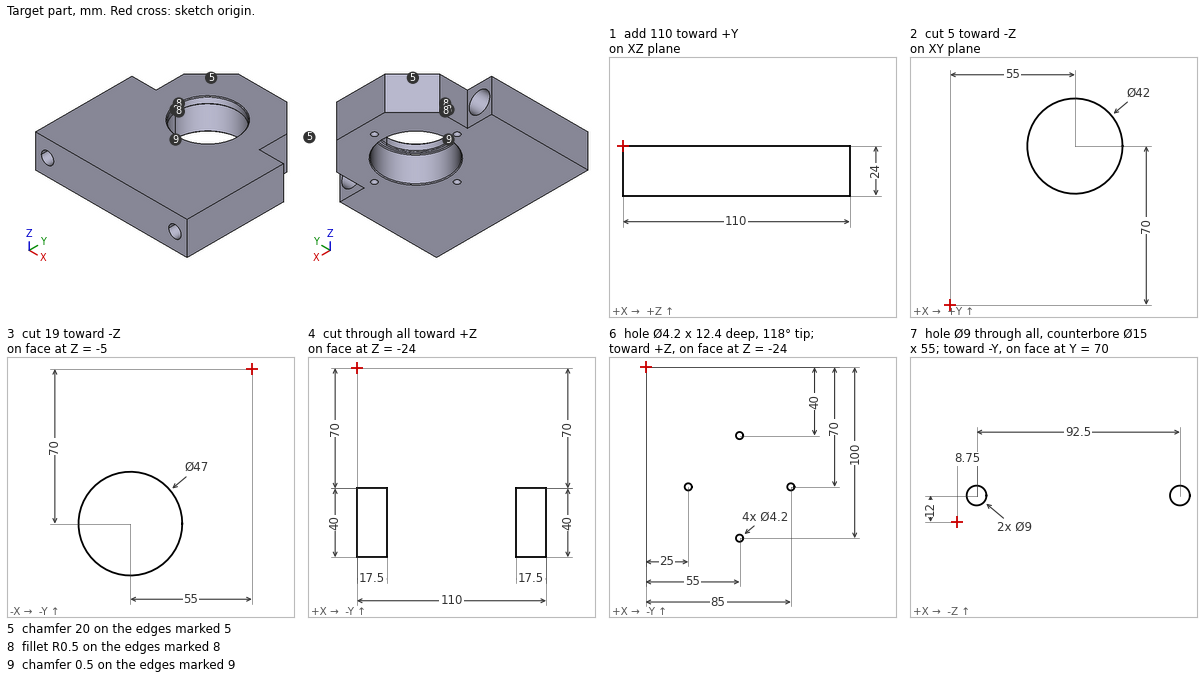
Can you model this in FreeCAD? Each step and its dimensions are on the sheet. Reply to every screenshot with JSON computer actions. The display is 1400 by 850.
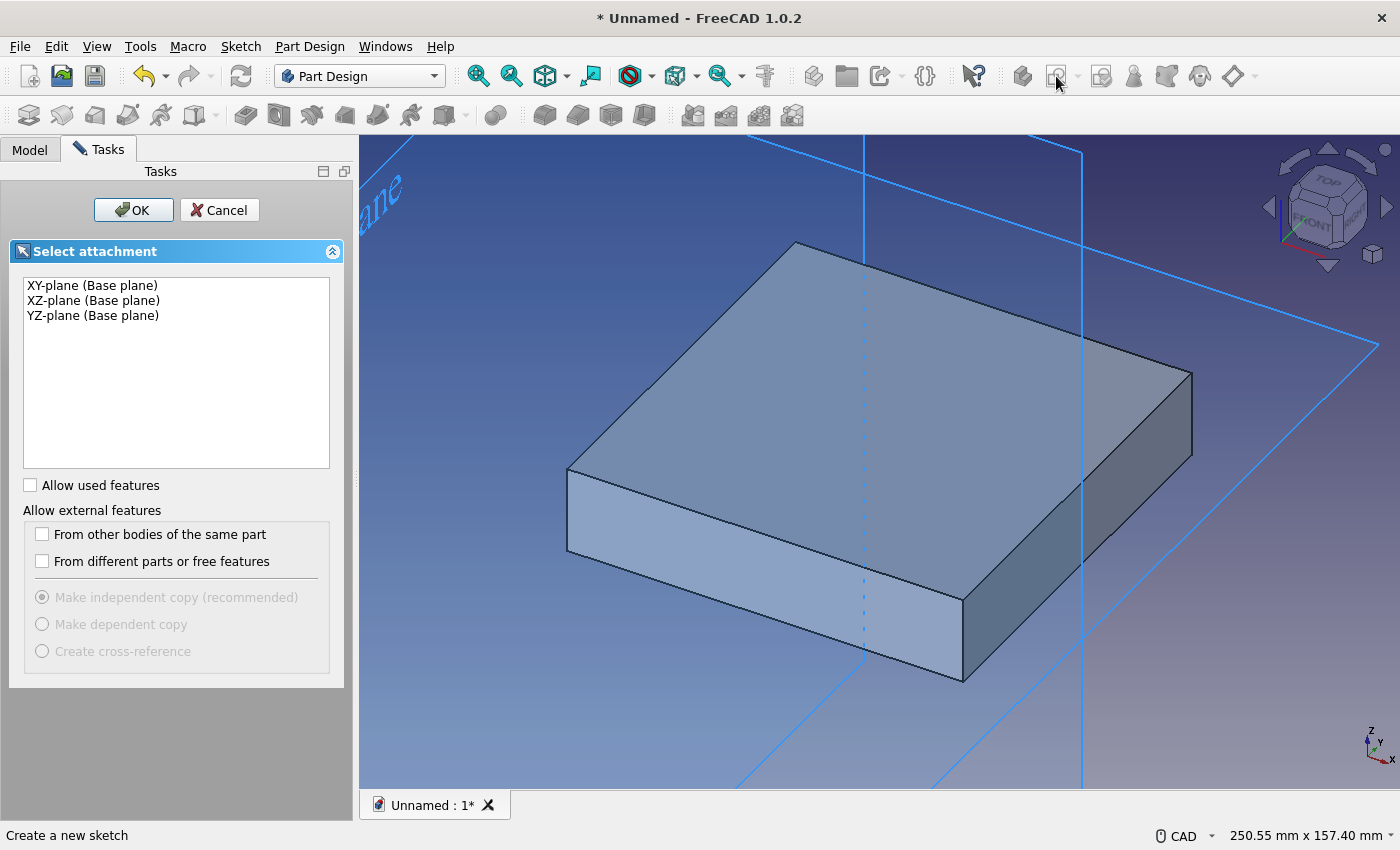
{"action": "left_click", "coordinate": [84, 286]}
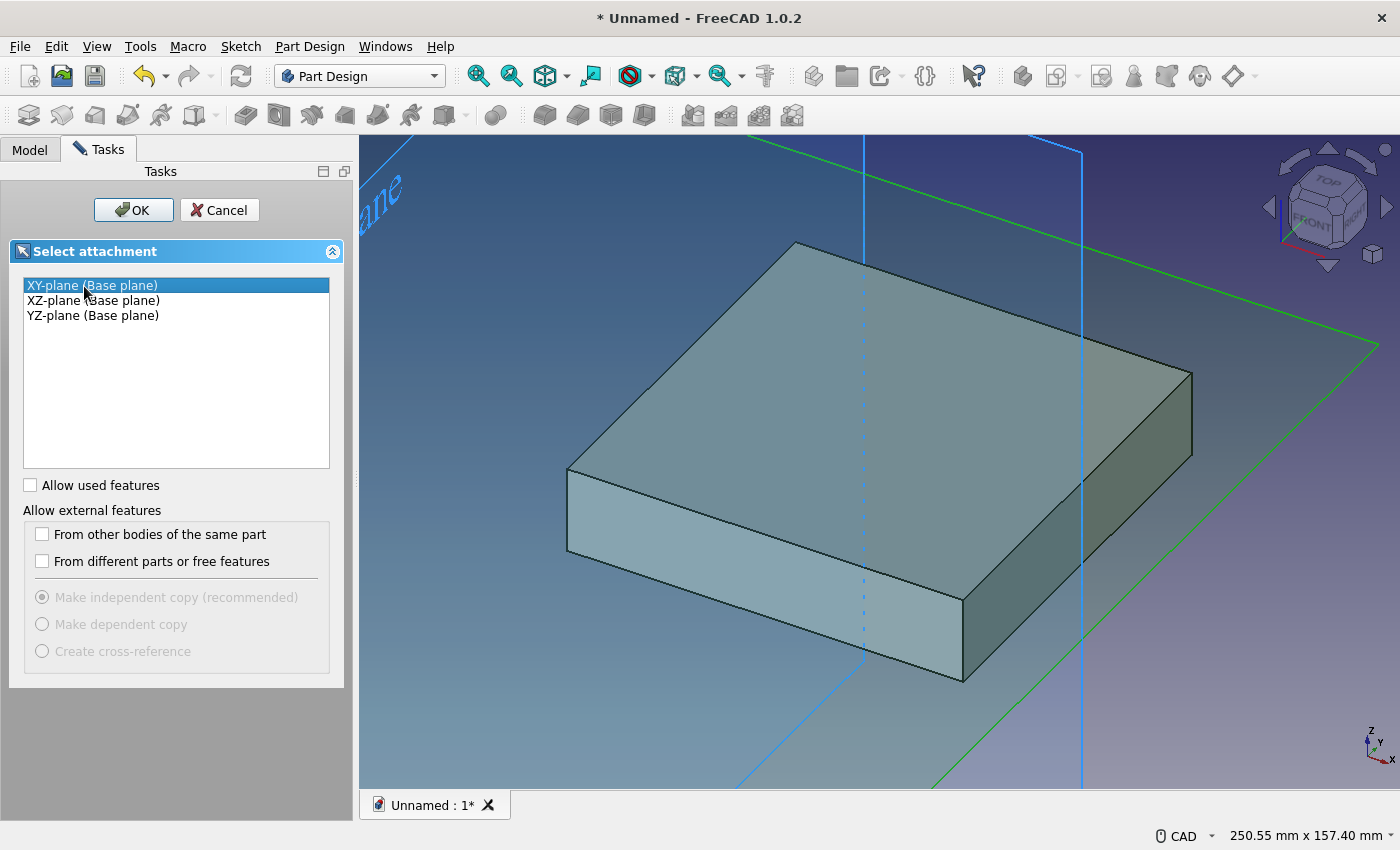
{"action": "left_click", "coordinate": [134, 210]}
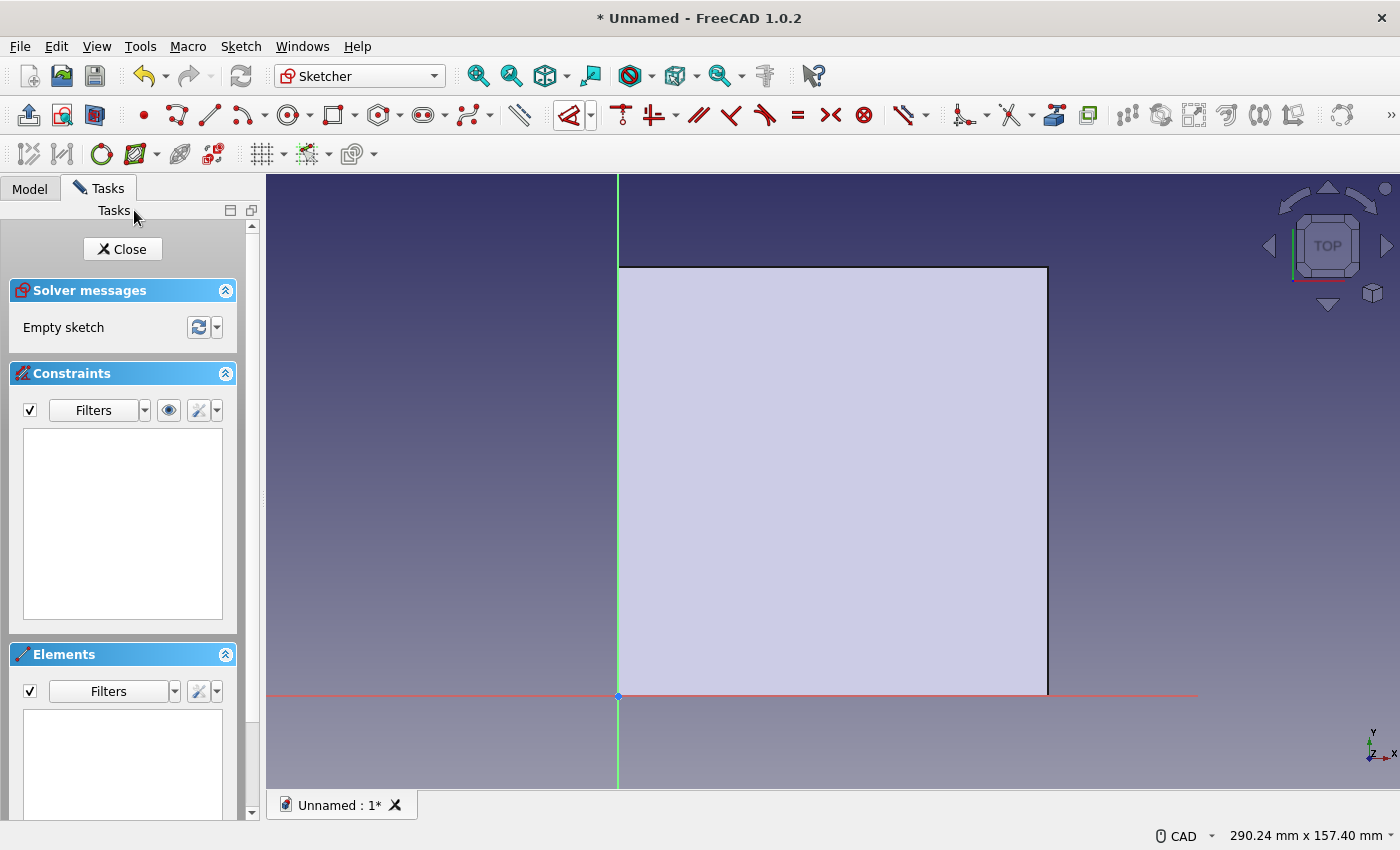
{"action": "left_click", "coordinate": [288, 116]}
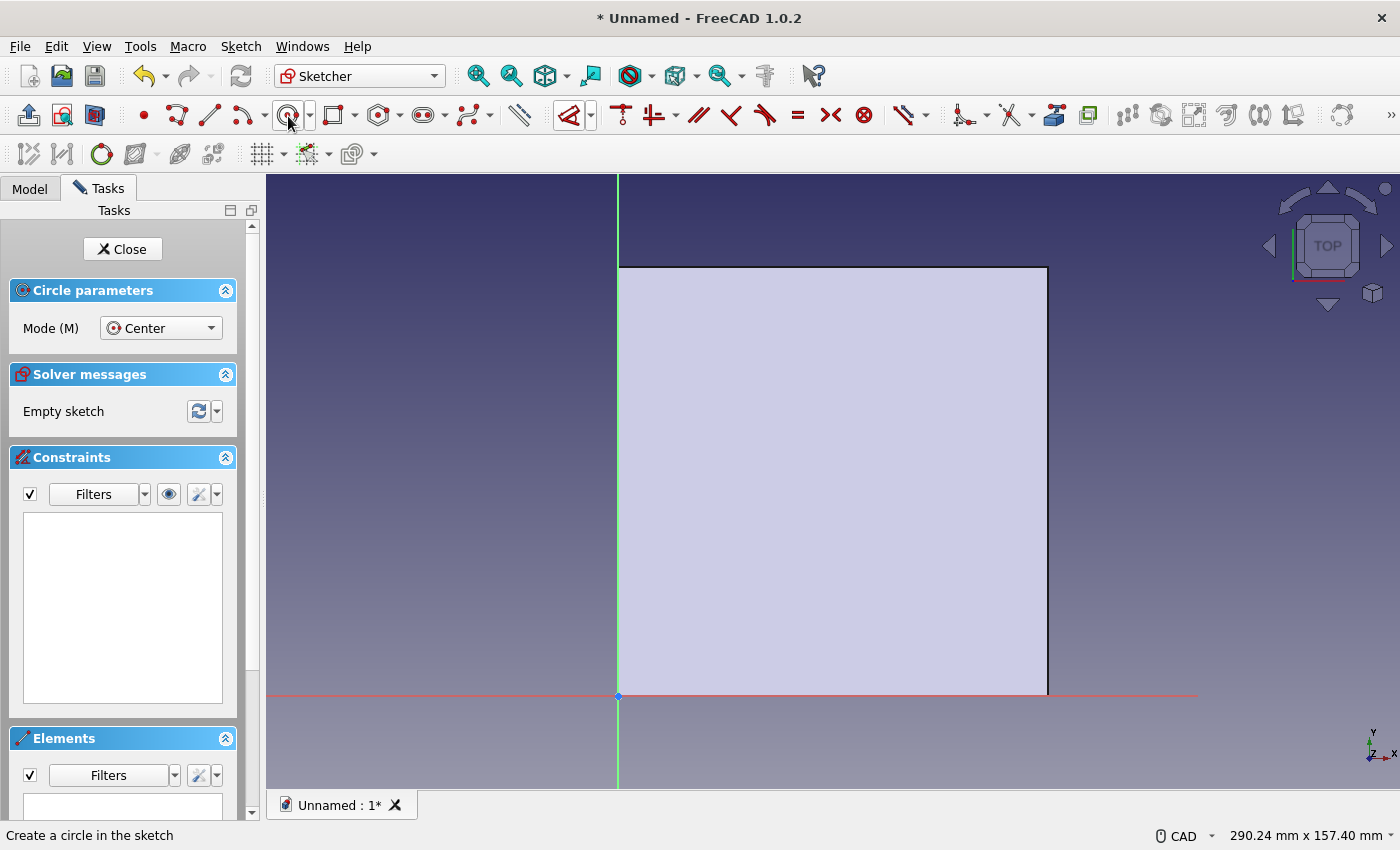
{"action": "left_click", "coordinate": [833, 423]}
{"action": "mouse_move", "coordinate": [891, 365]}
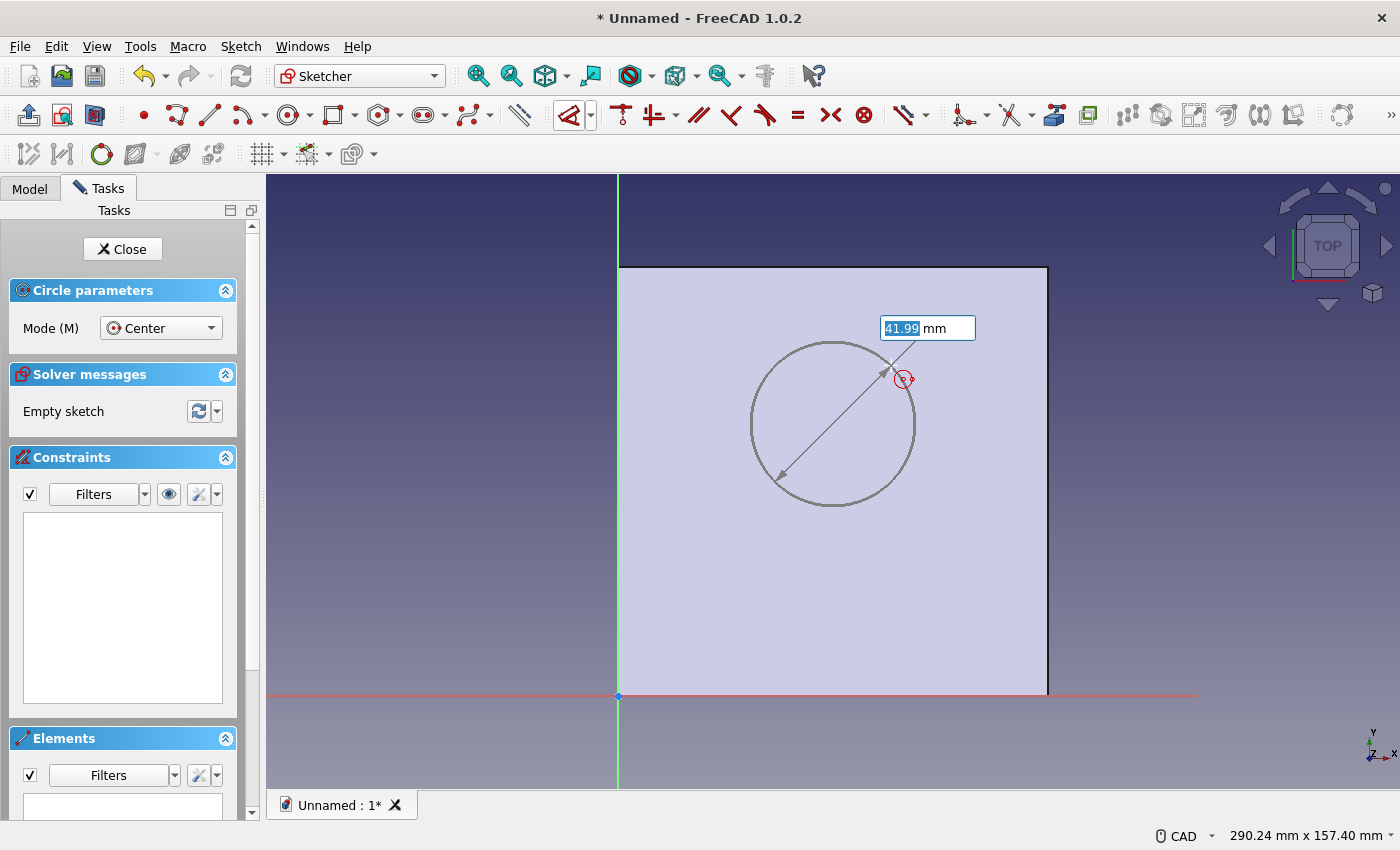
{"action": "type", "text": "42"}
{"action": "key", "text": "Return"}
{"action": "key", "text": "Escape"}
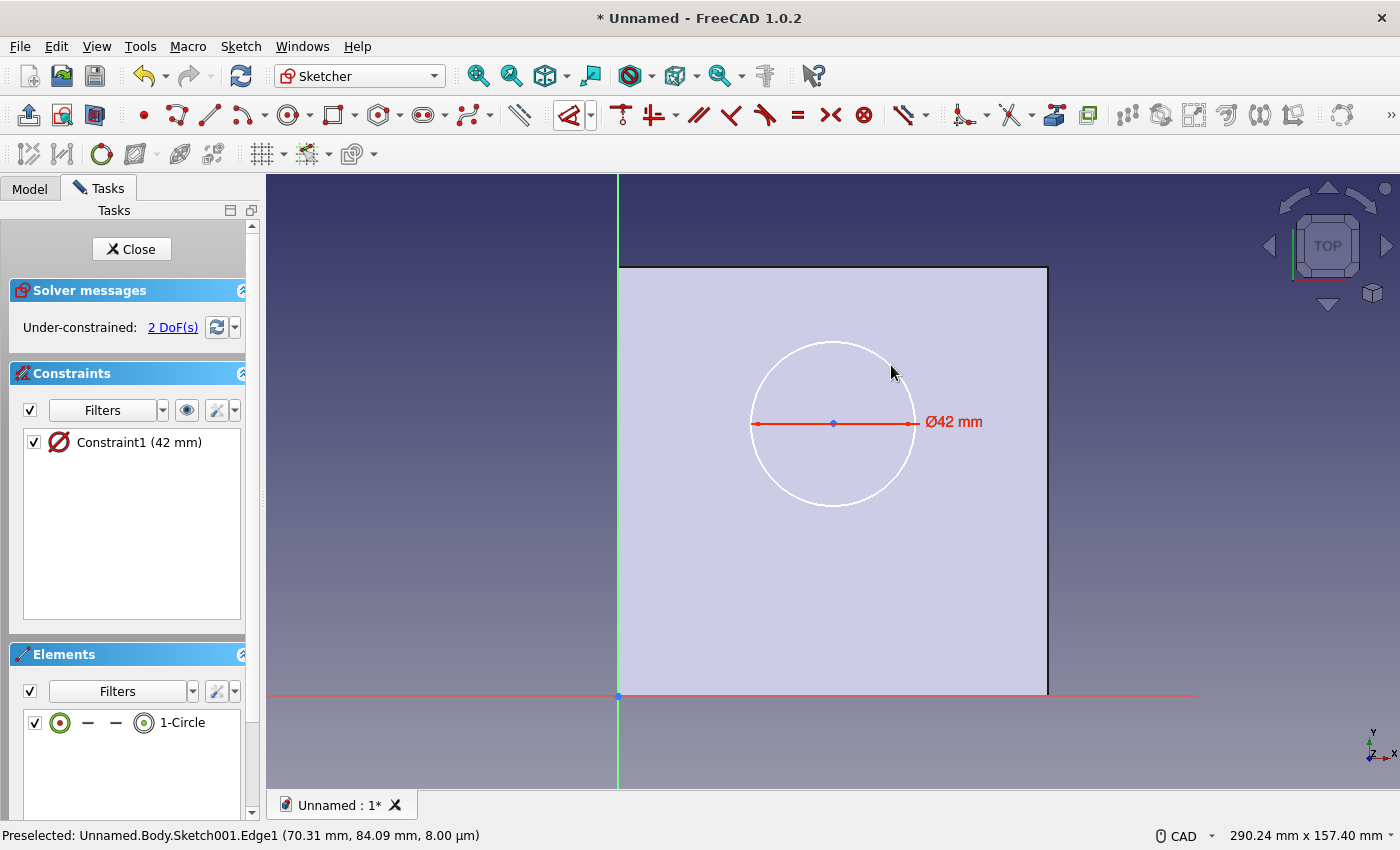
{"action": "left_click", "coordinate": [568, 116]}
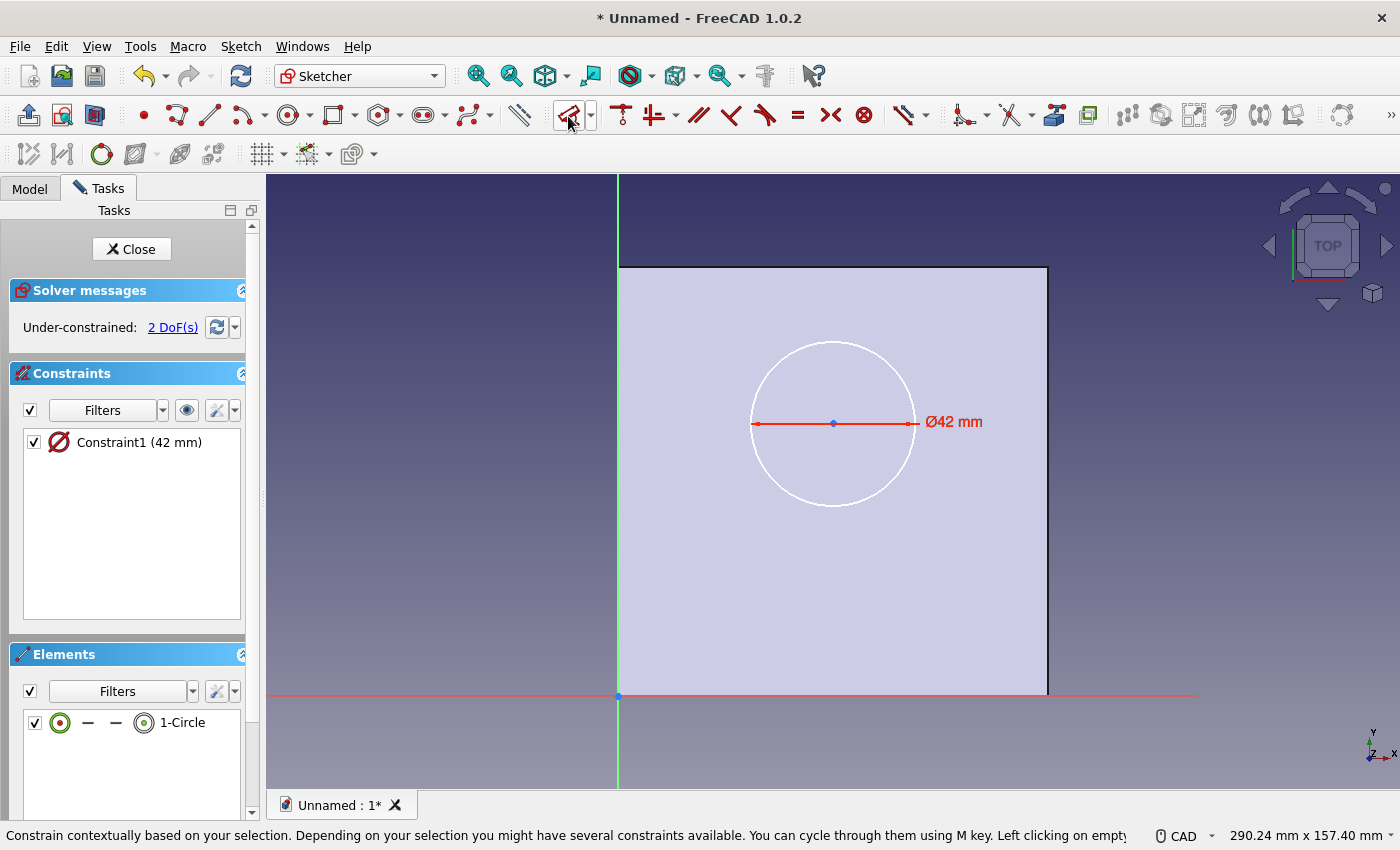
{"action": "left_click", "coordinate": [833, 424]}
{"action": "left_click", "coordinate": [726, 730]}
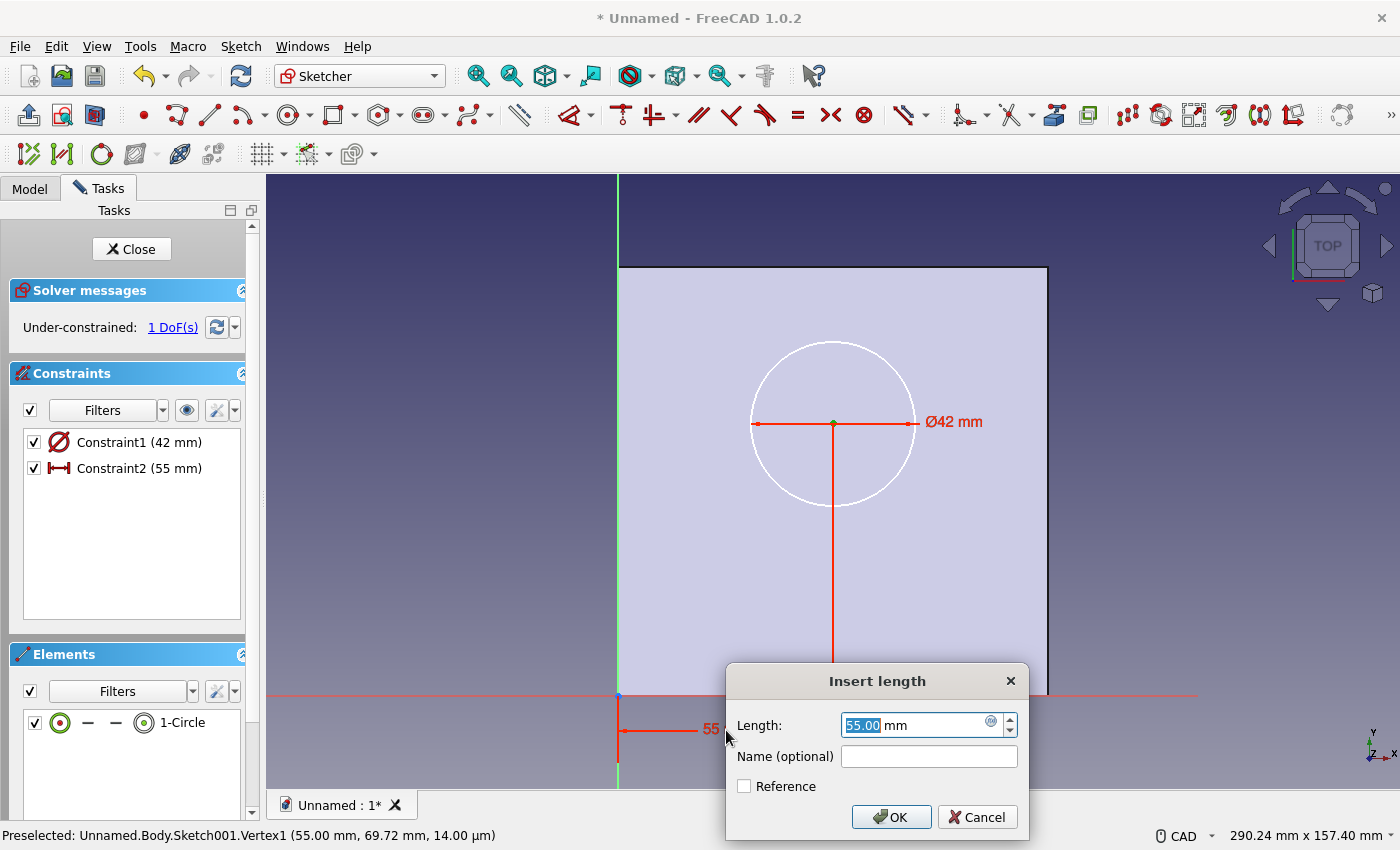
{"action": "type", "text": "55"}
{"action": "key", "text": "Return"}